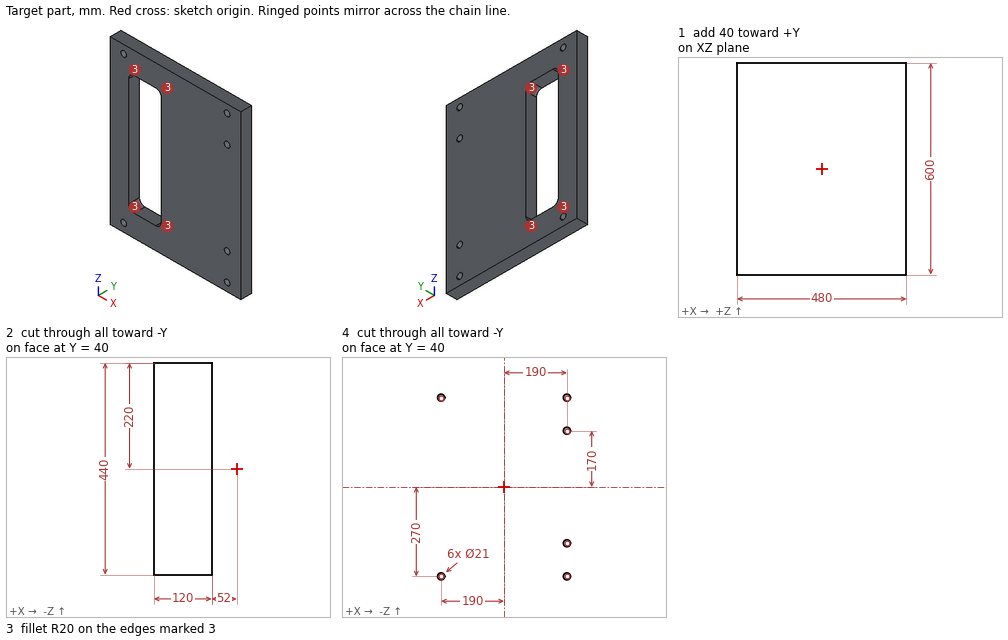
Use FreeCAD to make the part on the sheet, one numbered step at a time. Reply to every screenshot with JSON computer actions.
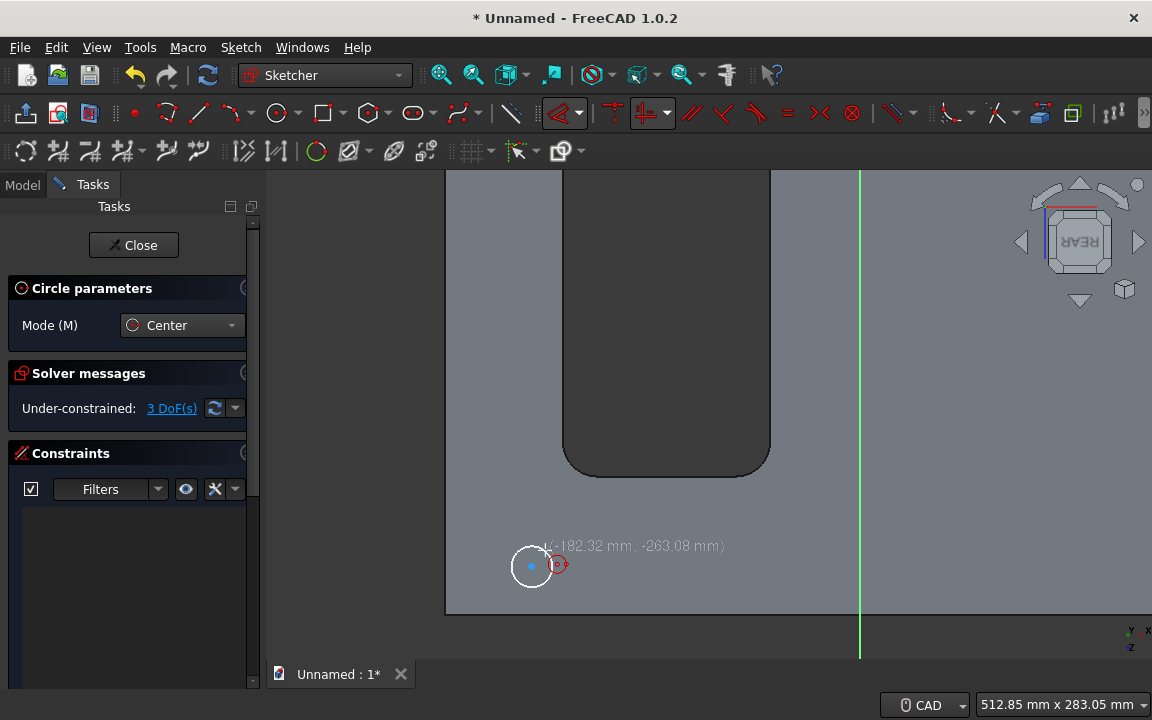
{"action": "scroll", "coordinate": [546, 552], "scroll_direction": "down", "scroll_amount": 6}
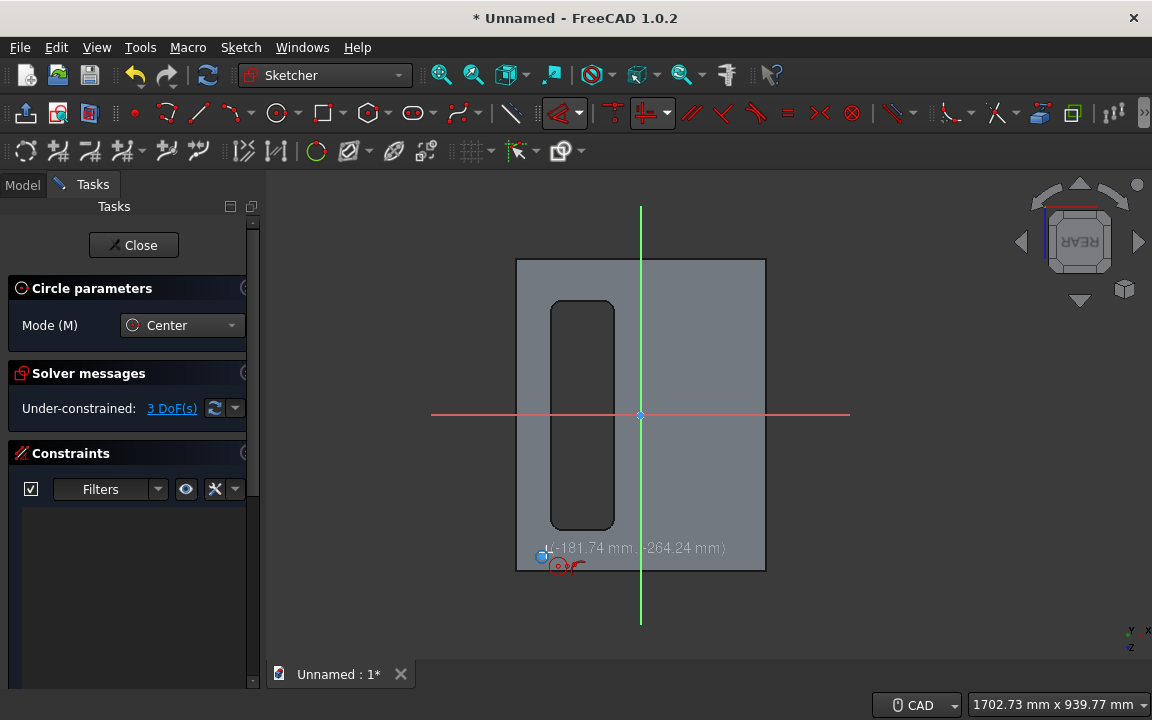
{"action": "scroll", "coordinate": [542, 275], "scroll_direction": "up", "scroll_amount": 8}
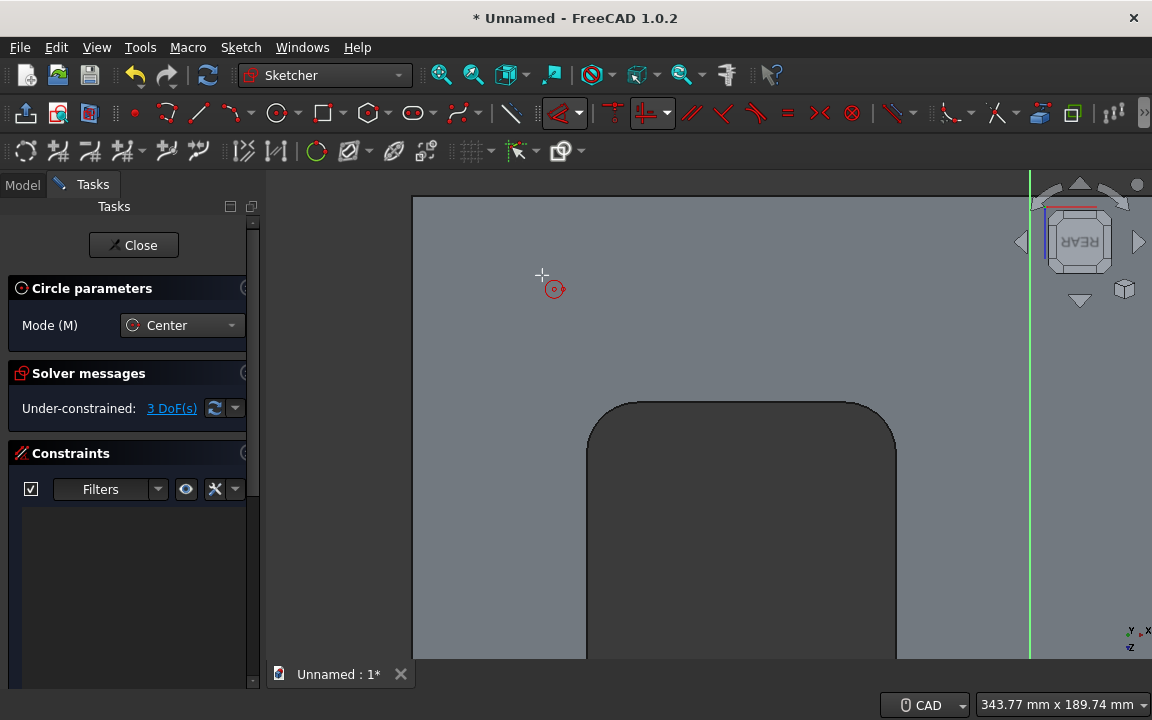
{"action": "scroll", "coordinate": [542, 274], "scroll_direction": "down", "scroll_amount": 8}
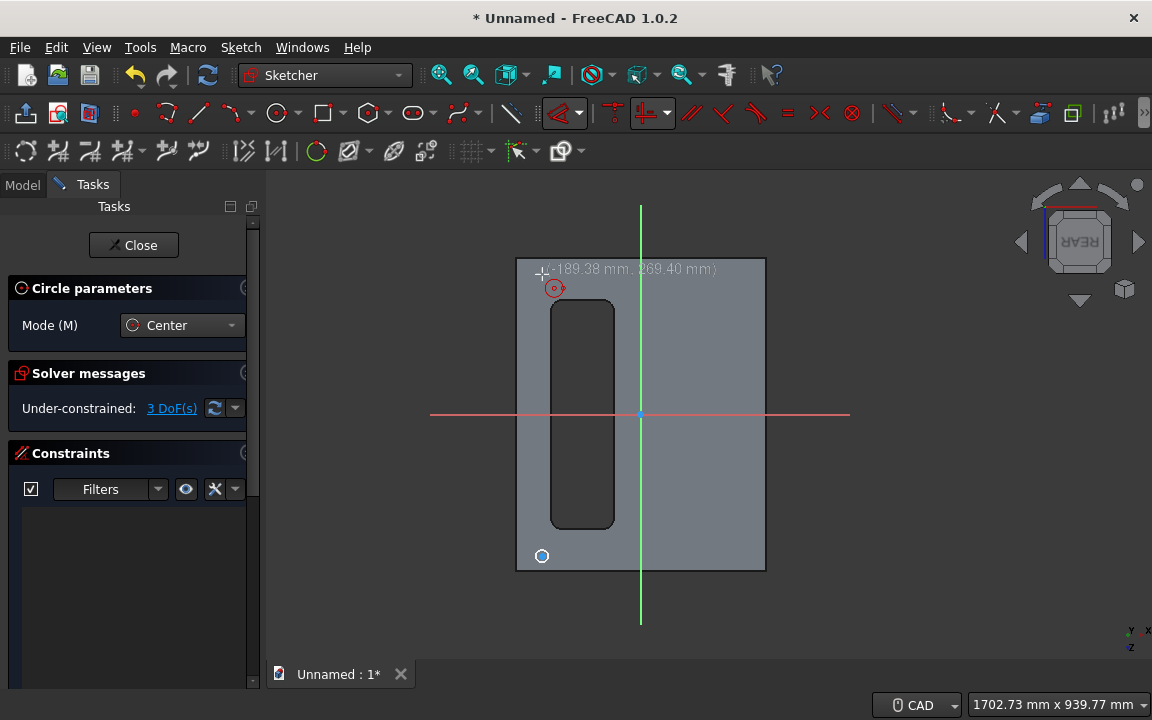
{"action": "left_click", "coordinate": [542, 274]}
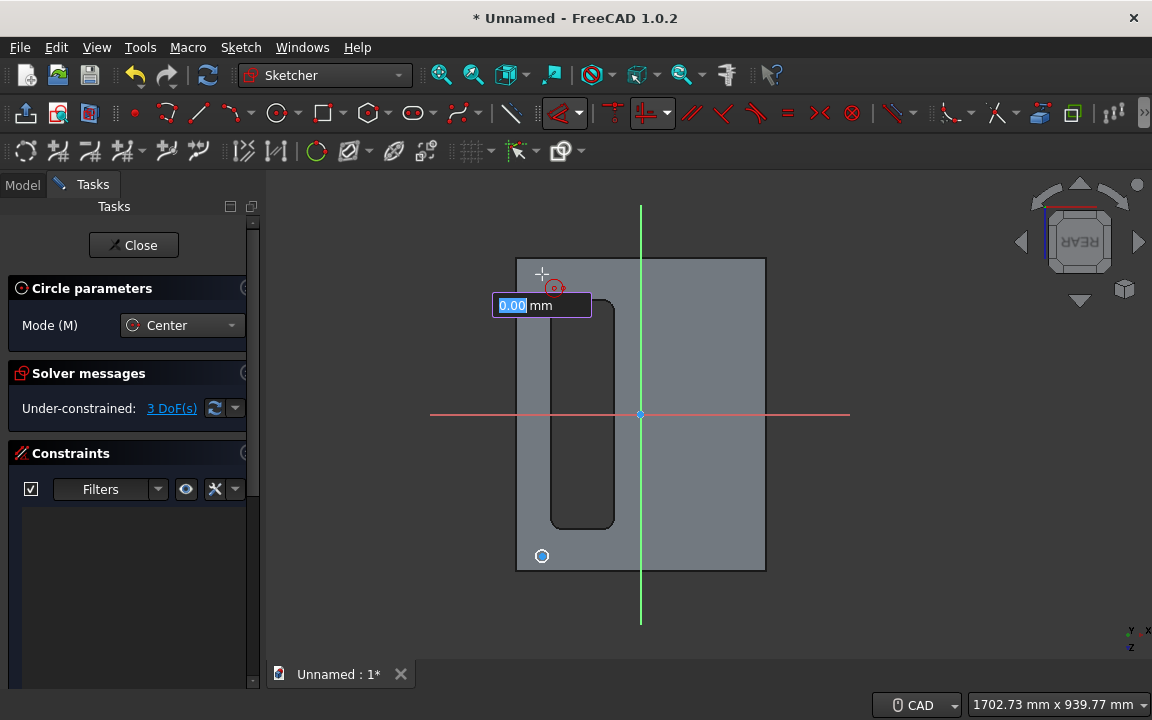
{"action": "scroll", "coordinate": [546, 270], "scroll_direction": "up", "scroll_amount": 6}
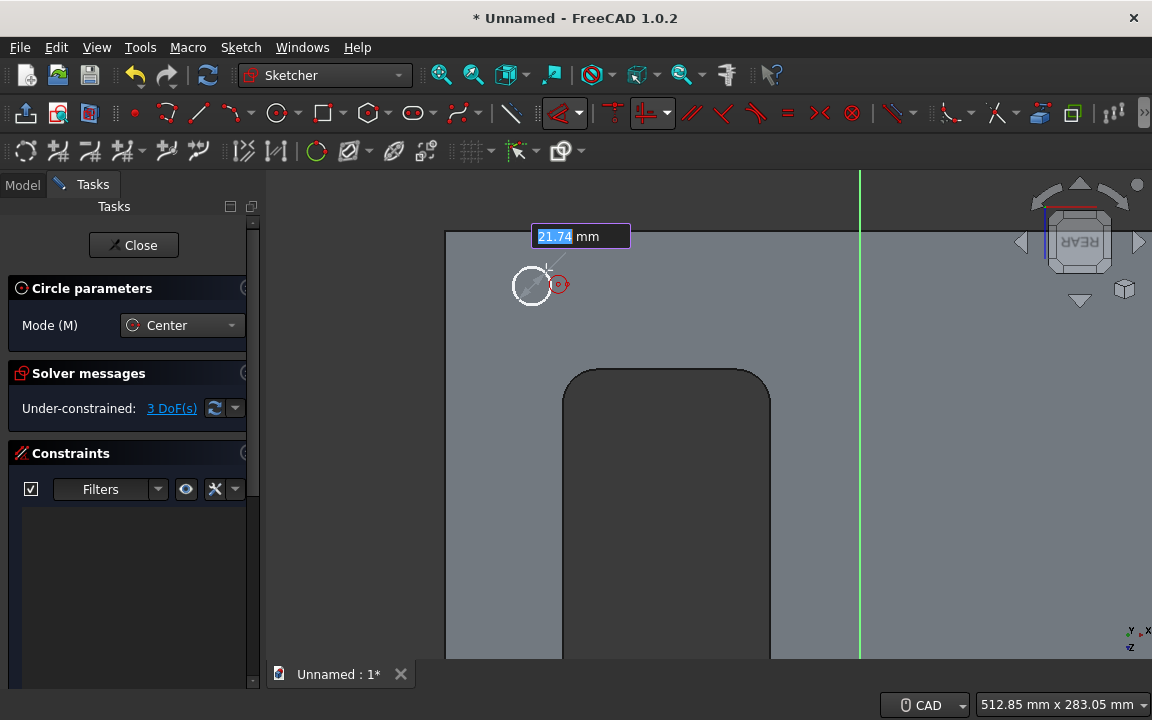
{"action": "left_click", "coordinate": [545, 270]}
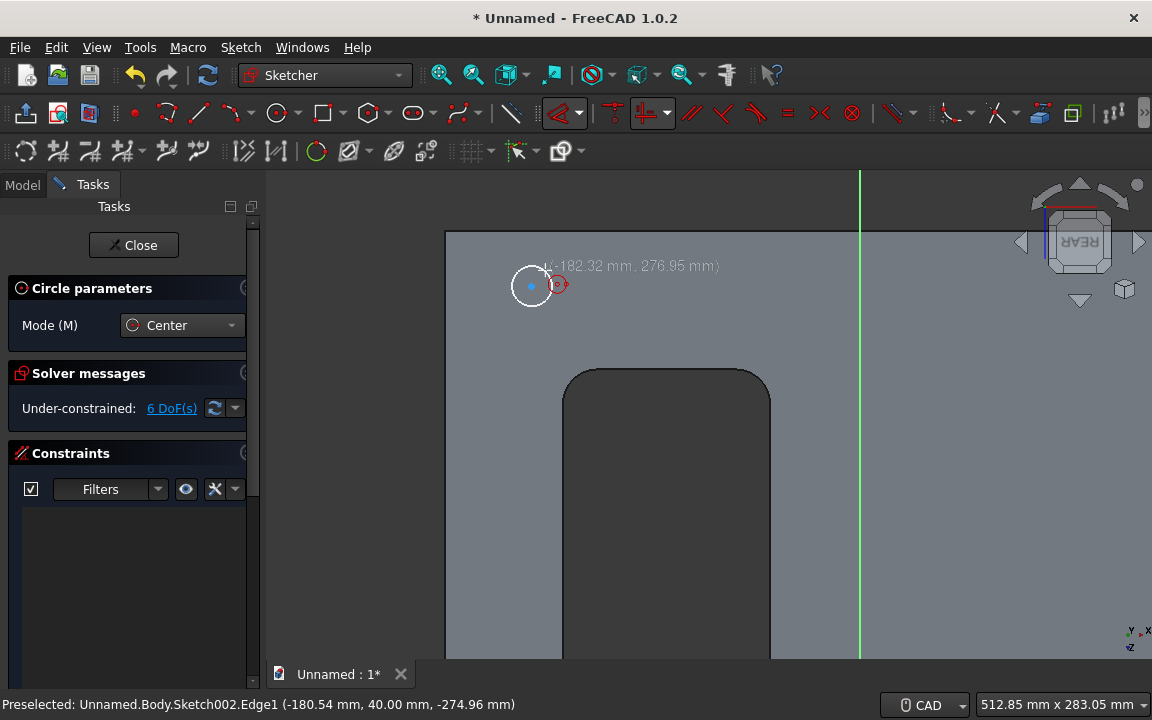
{"action": "scroll", "coordinate": [546, 270], "scroll_direction": "down", "scroll_amount": 6}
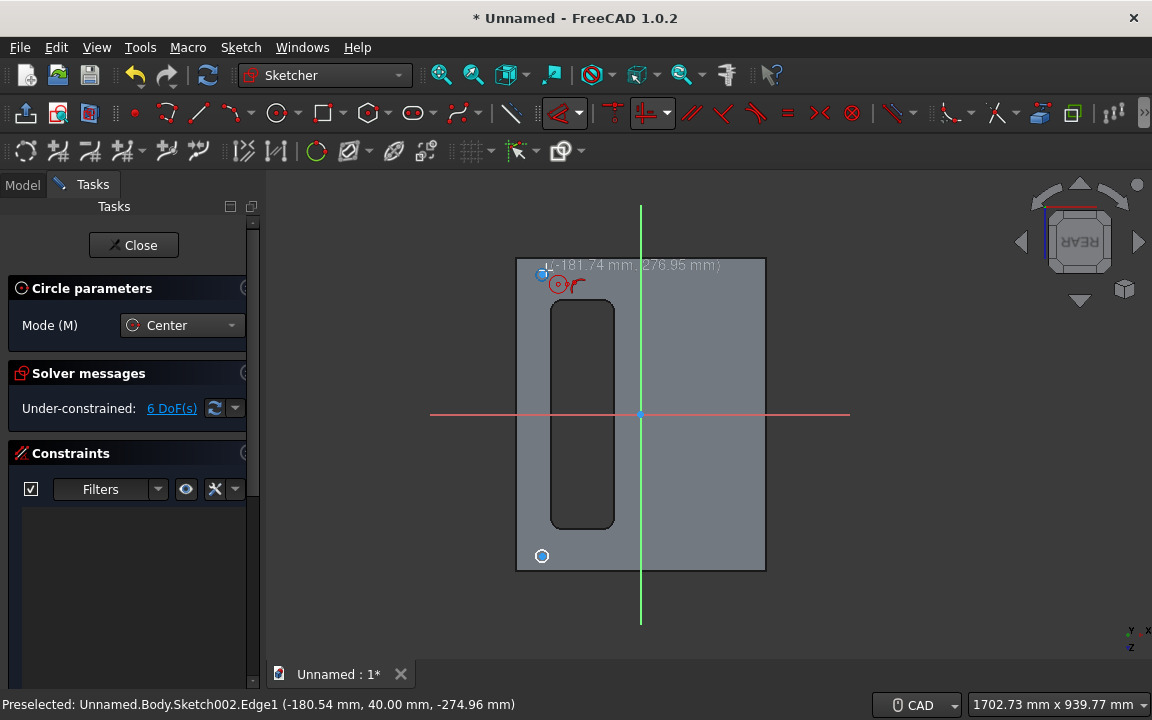
{"action": "scroll", "coordinate": [740, 274], "scroll_direction": "up", "scroll_amount": 8}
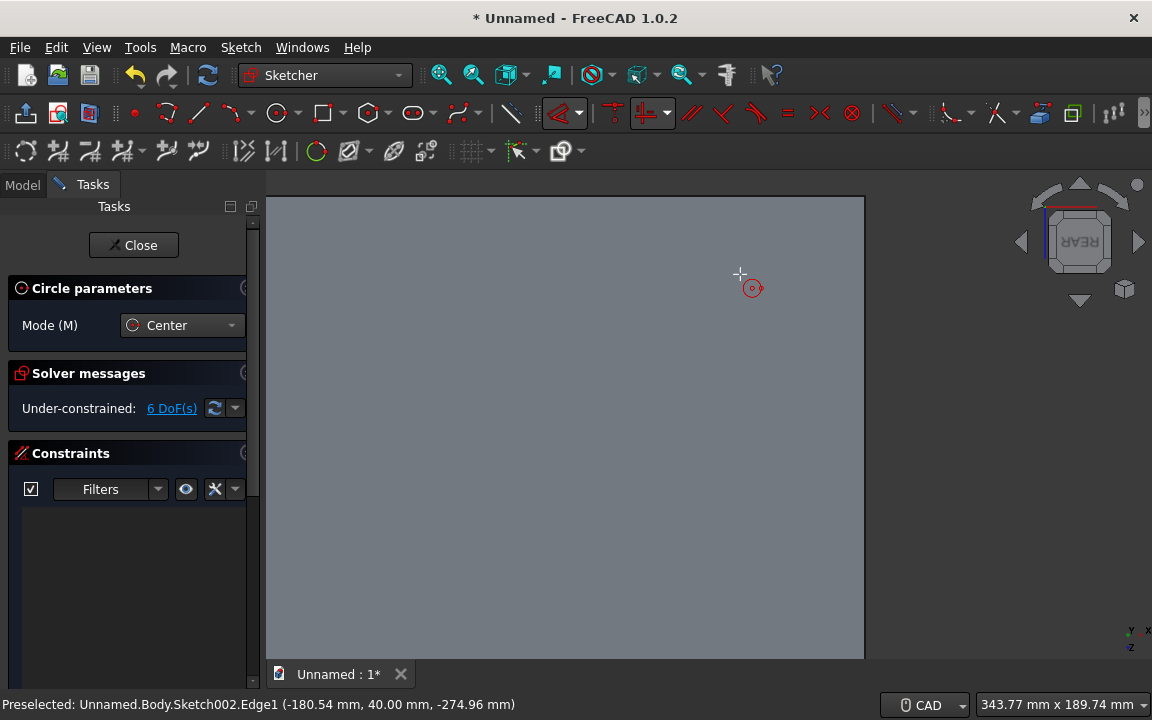
{"action": "scroll", "coordinate": [740, 274], "scroll_direction": "down", "scroll_amount": 8}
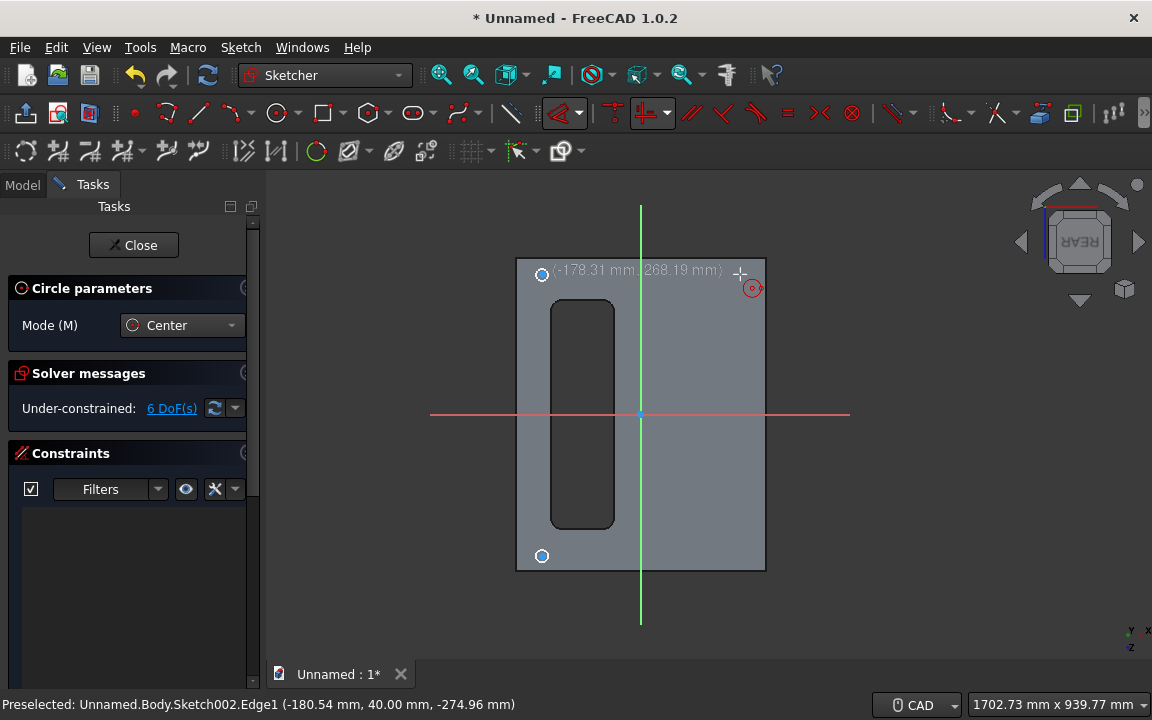
{"action": "left_click", "coordinate": [740, 274]}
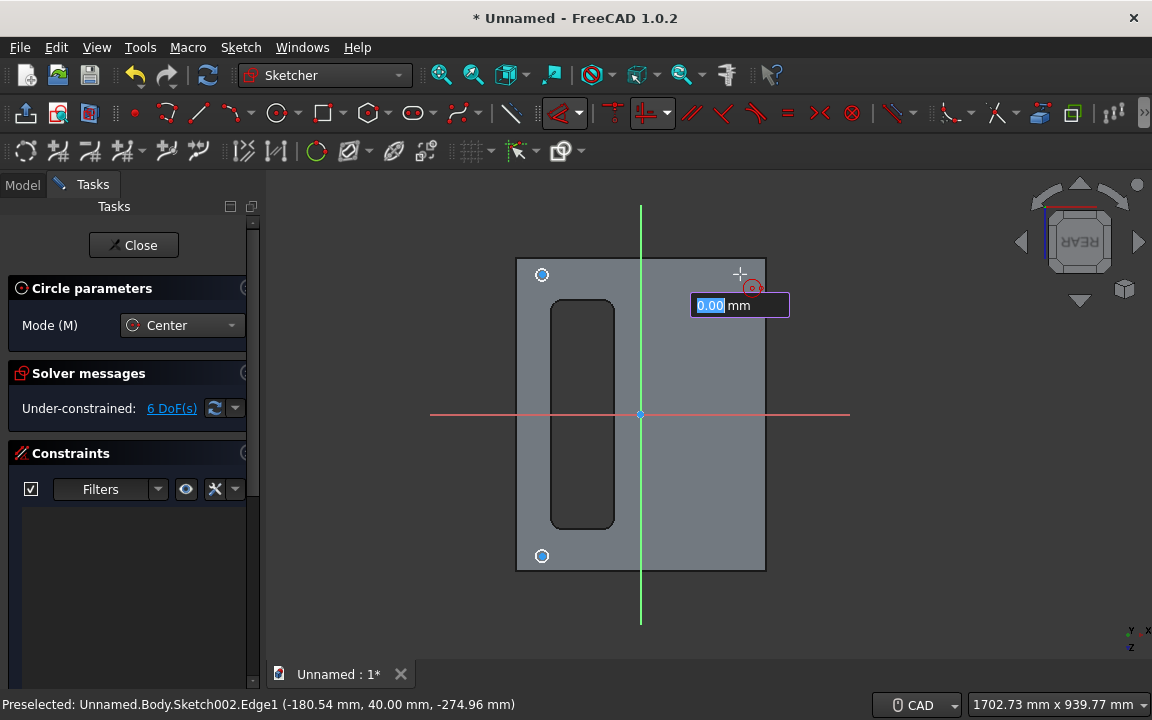
{"action": "scroll", "coordinate": [744, 270], "scroll_direction": "up", "scroll_amount": 6}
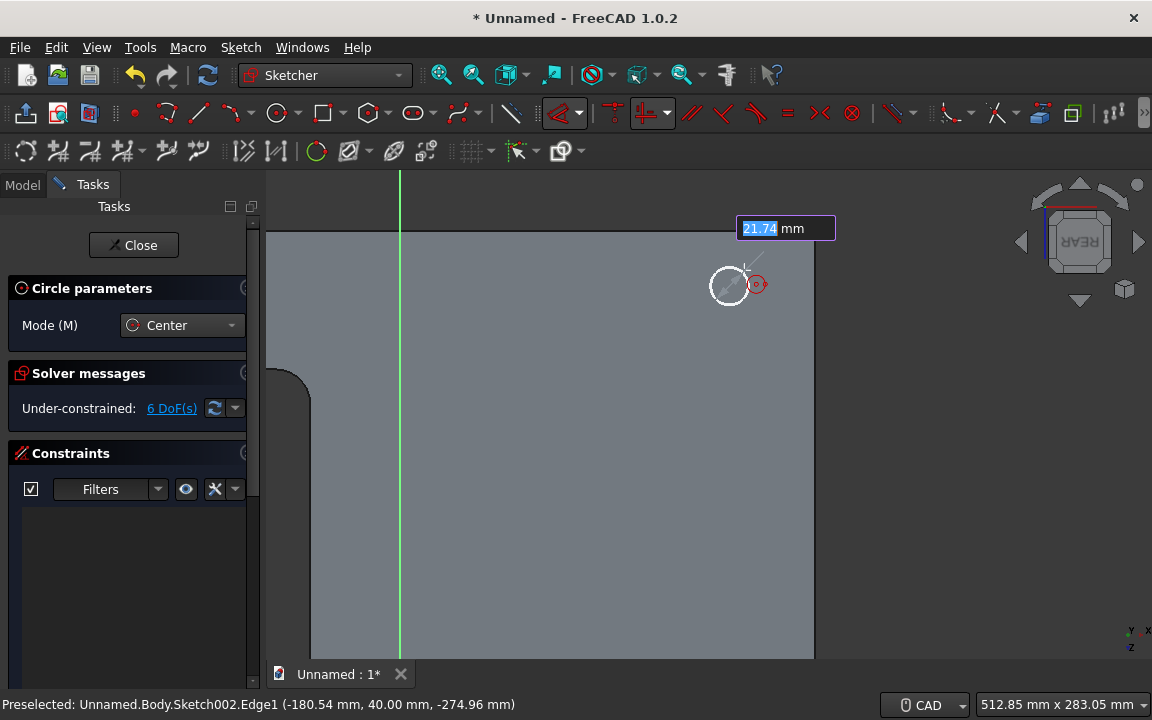
{"action": "left_click", "coordinate": [741, 270]}